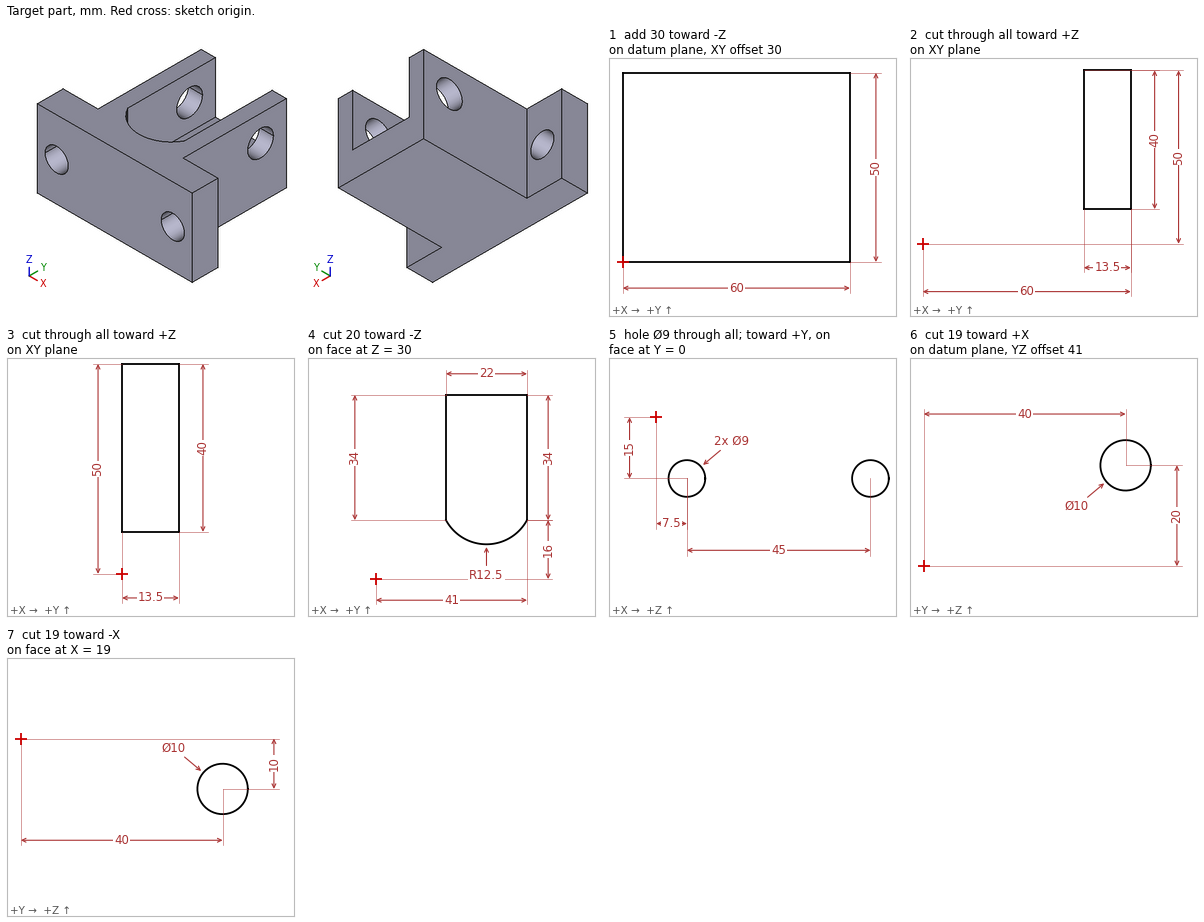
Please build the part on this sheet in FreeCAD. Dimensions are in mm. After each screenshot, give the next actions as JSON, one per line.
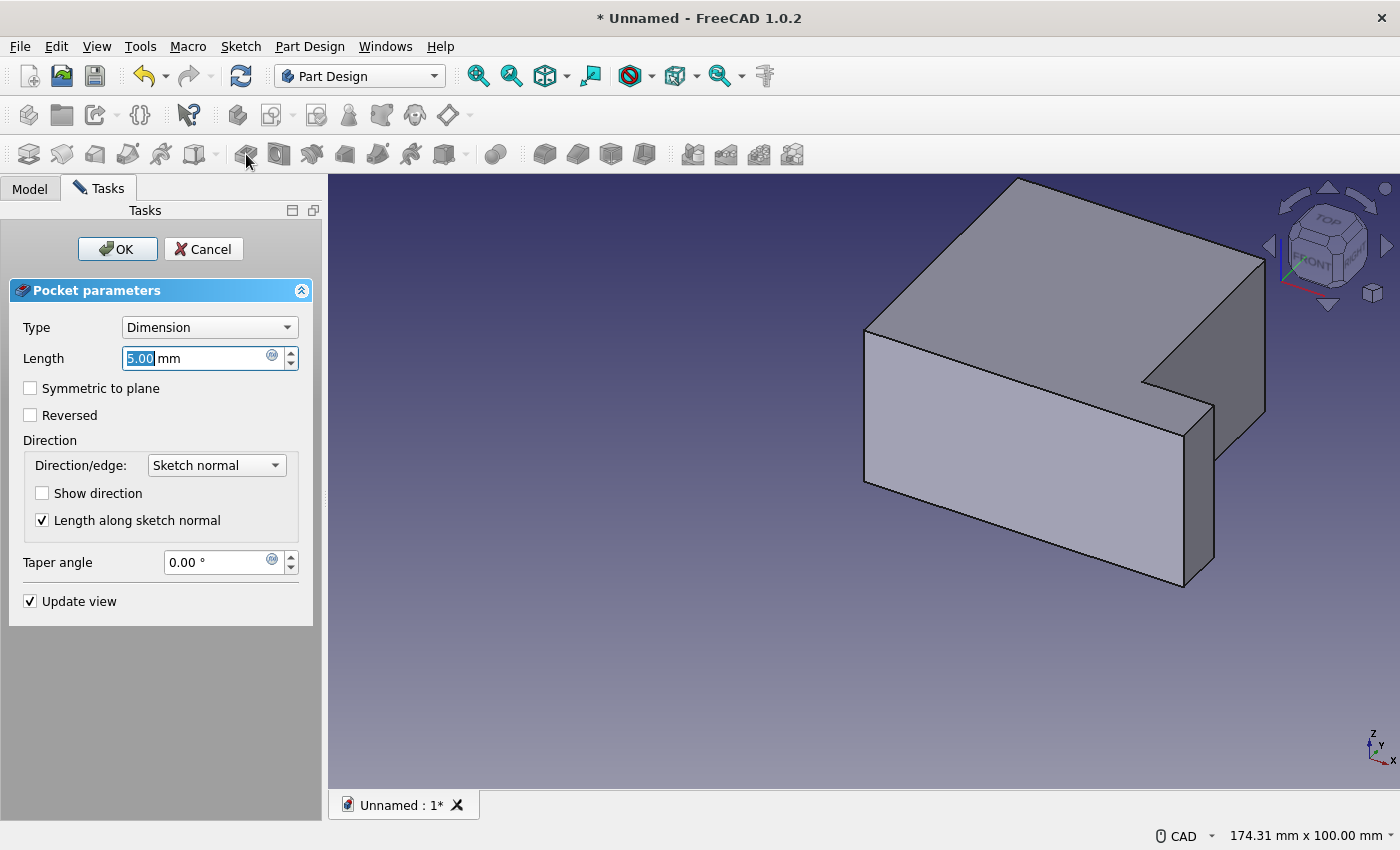
{"action": "left_click", "coordinate": [210, 328]}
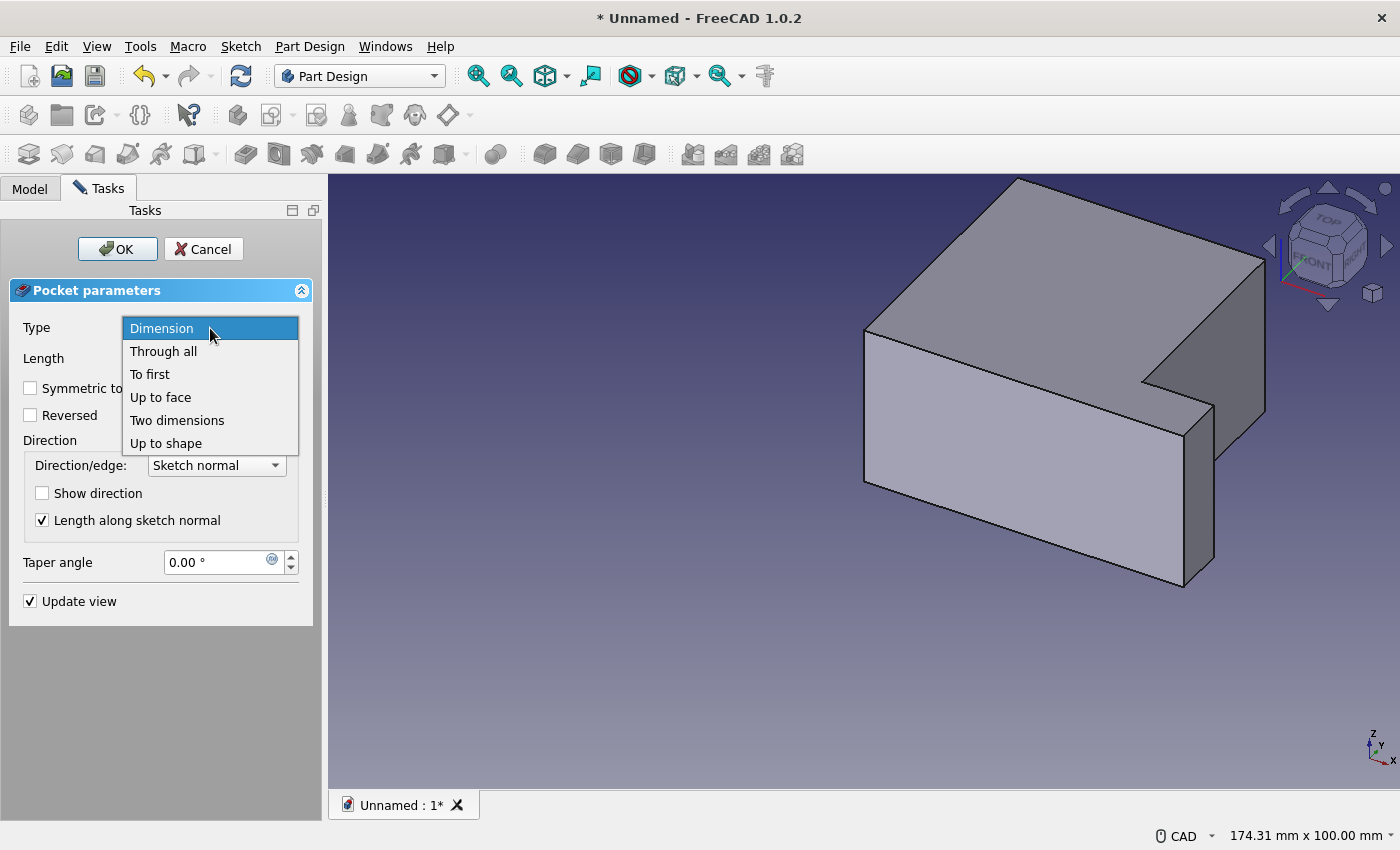
{"action": "left_click", "coordinate": [208, 352]}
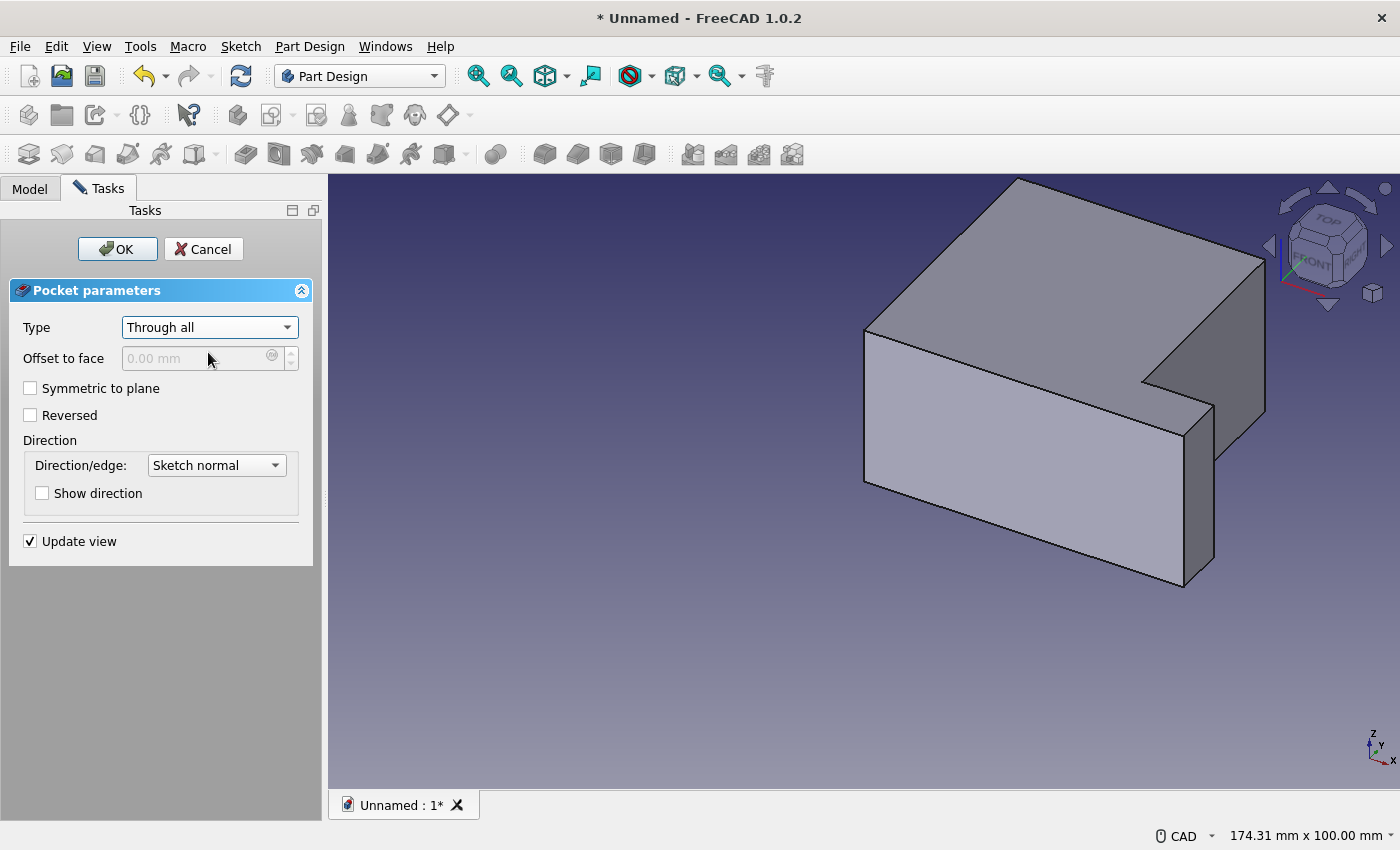
{"action": "left_click", "coordinate": [31, 415]}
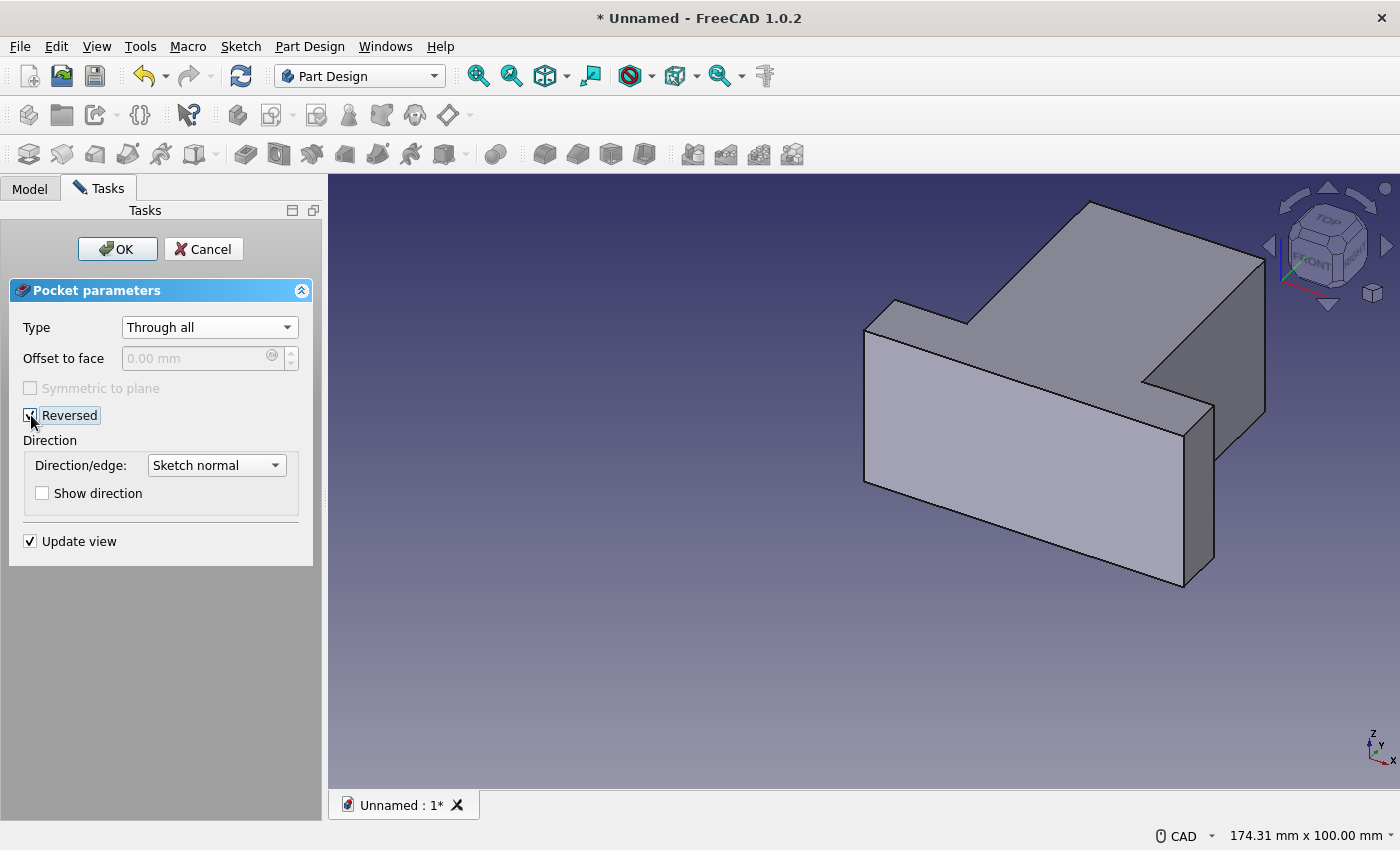
{"action": "left_click", "coordinate": [118, 249]}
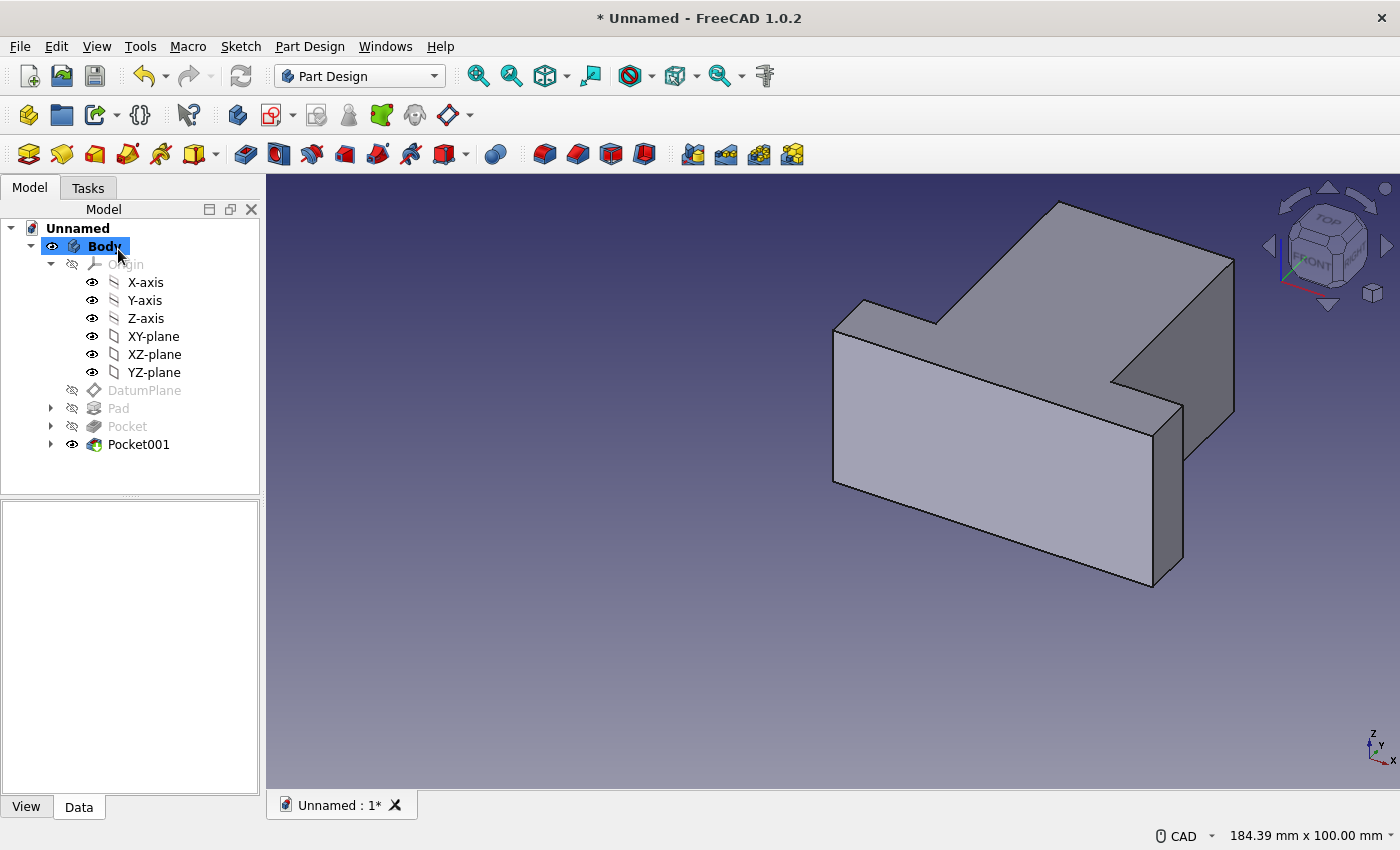
{"action": "left_click", "coordinate": [1092, 284]}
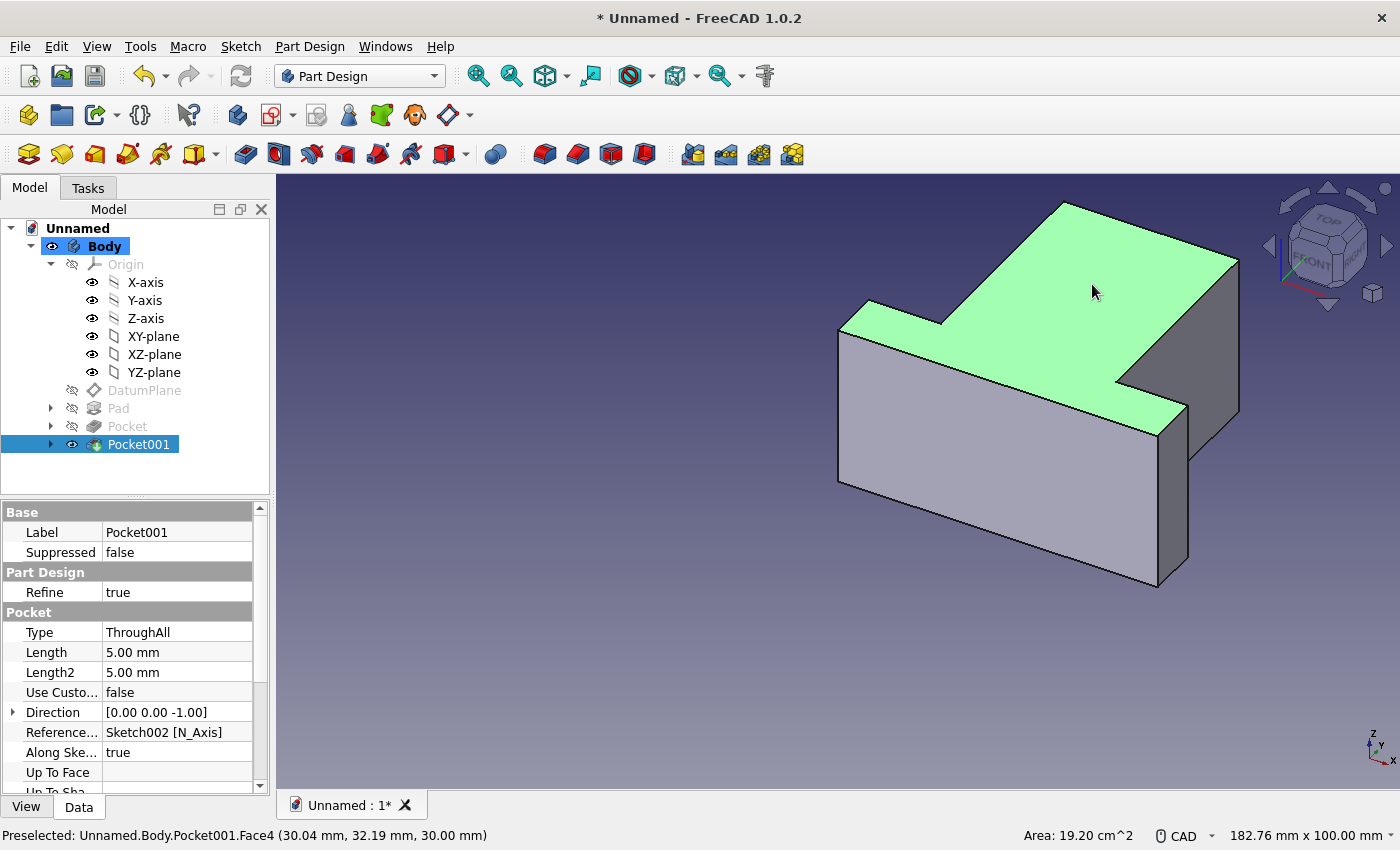
{"action": "left_click", "coordinate": [270, 116]}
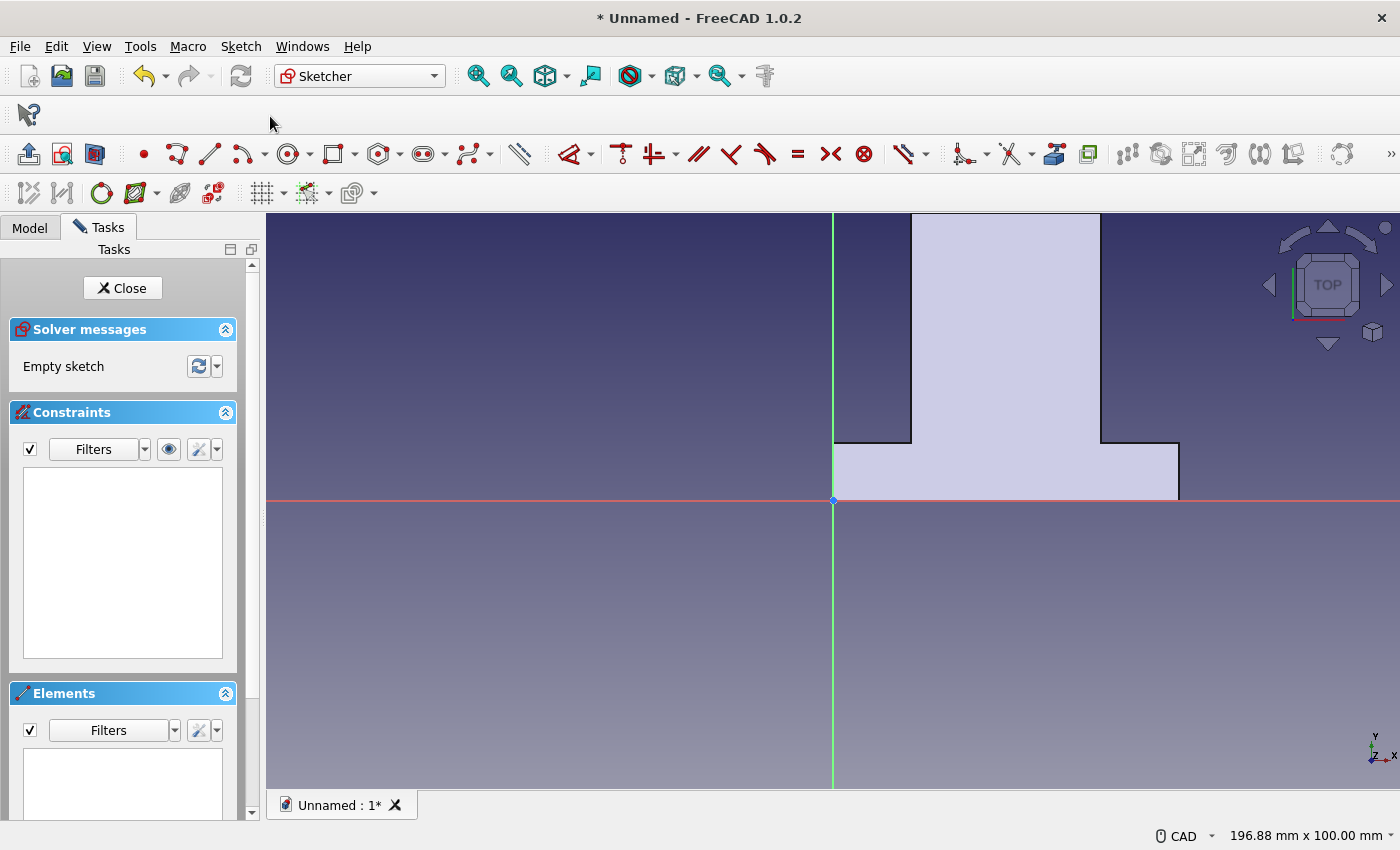
{"action": "scroll", "coordinate": [294, 761], "scroll_direction": "down", "scroll_amount": 1}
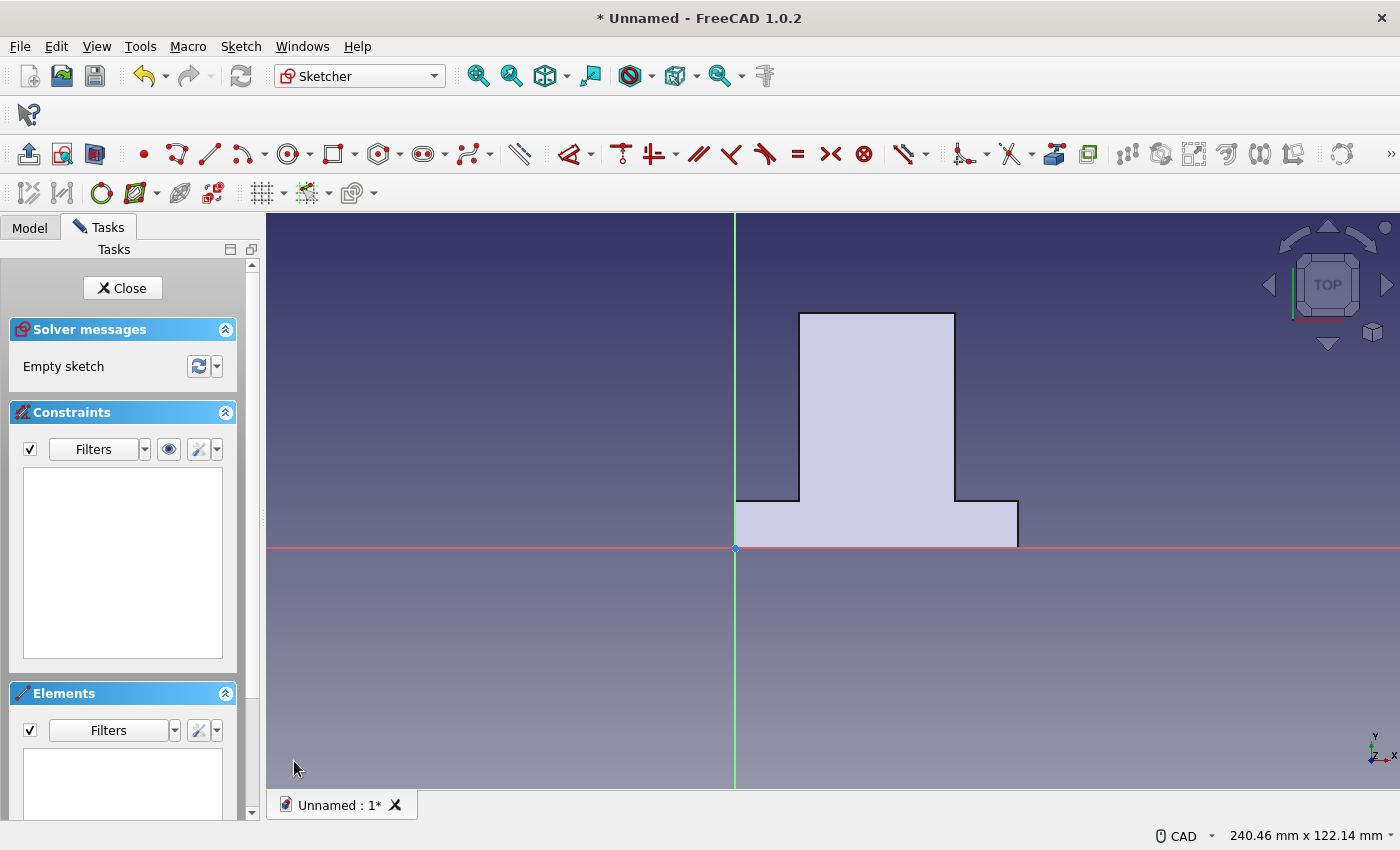
{"action": "scroll", "coordinate": [969, 287], "scroll_direction": "up", "scroll_amount": 2}